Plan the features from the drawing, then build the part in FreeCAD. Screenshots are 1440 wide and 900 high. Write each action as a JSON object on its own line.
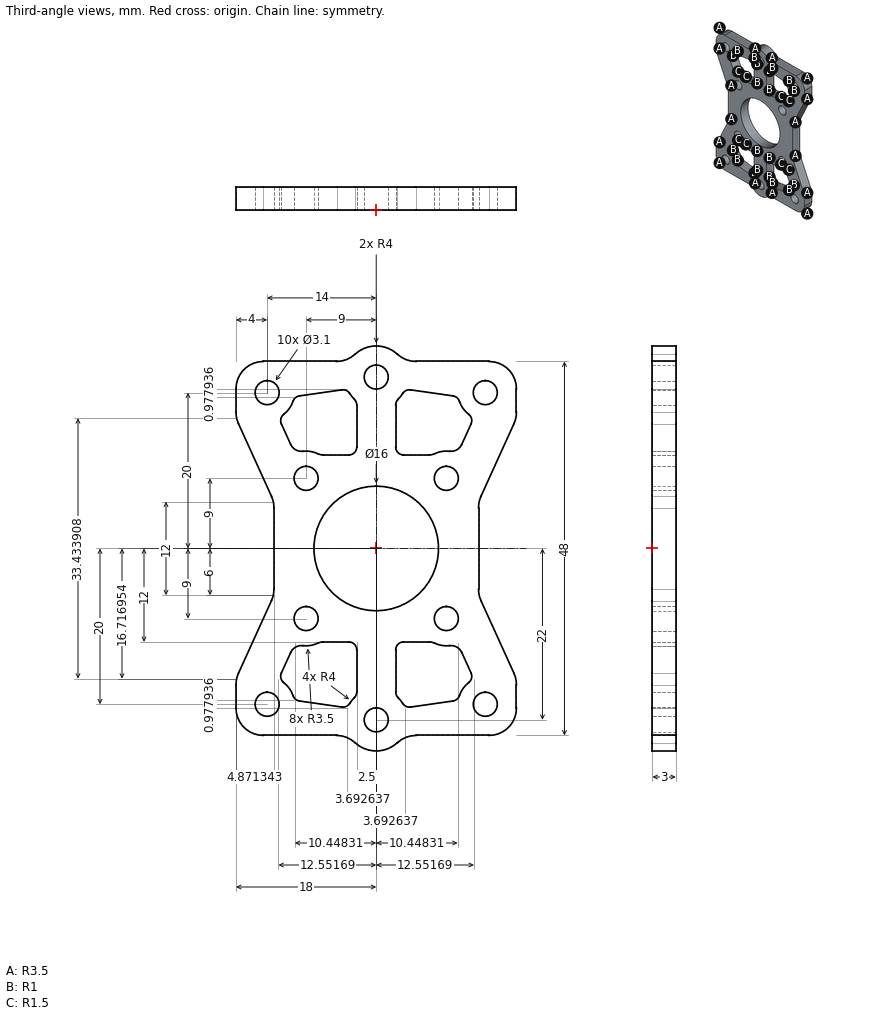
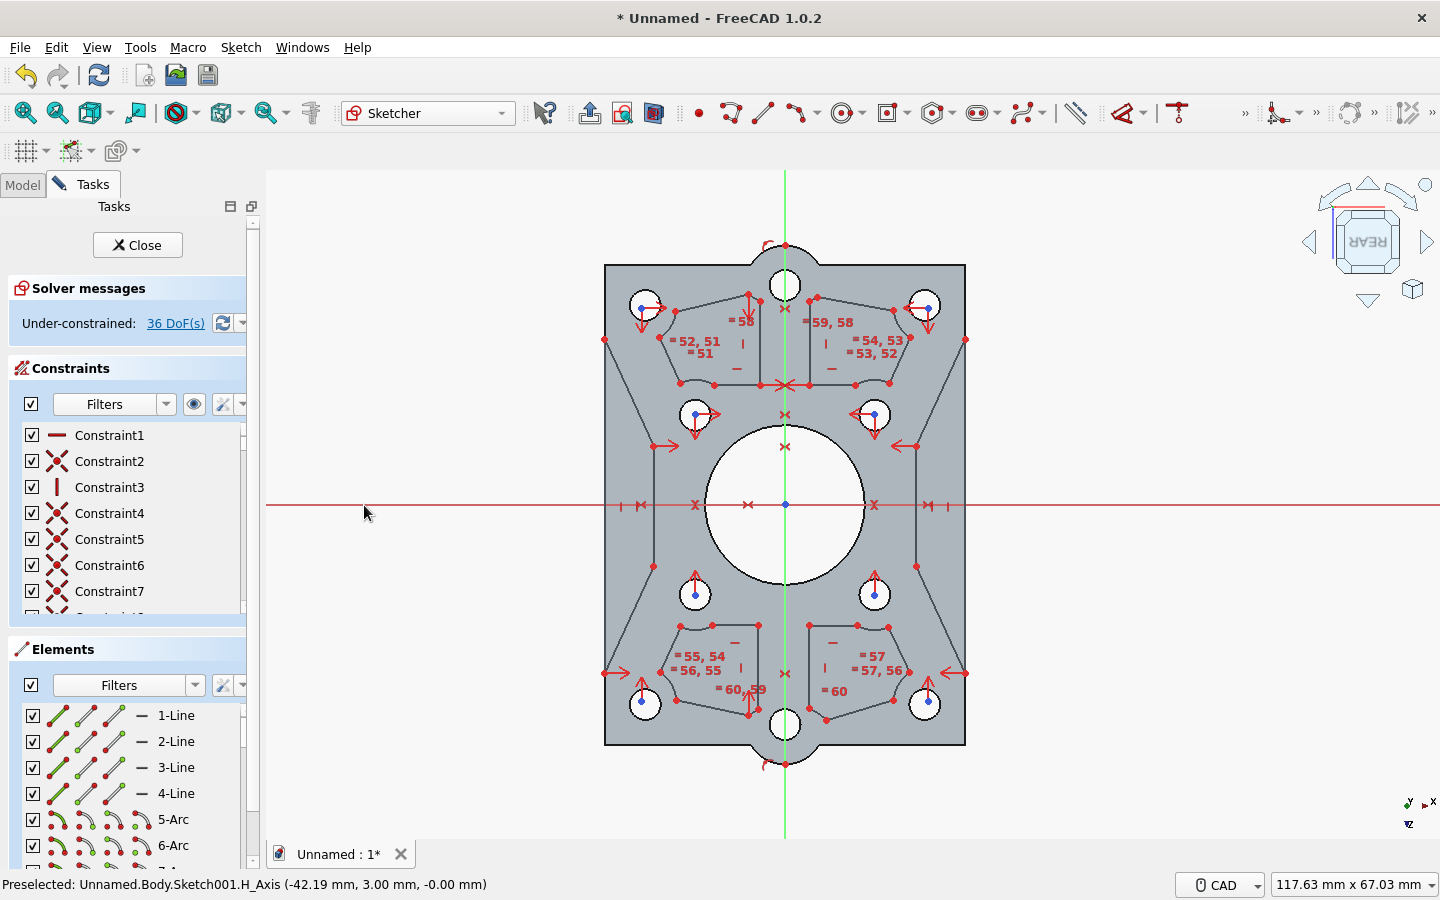
{"action": "left_click", "coordinate": [760, 385]}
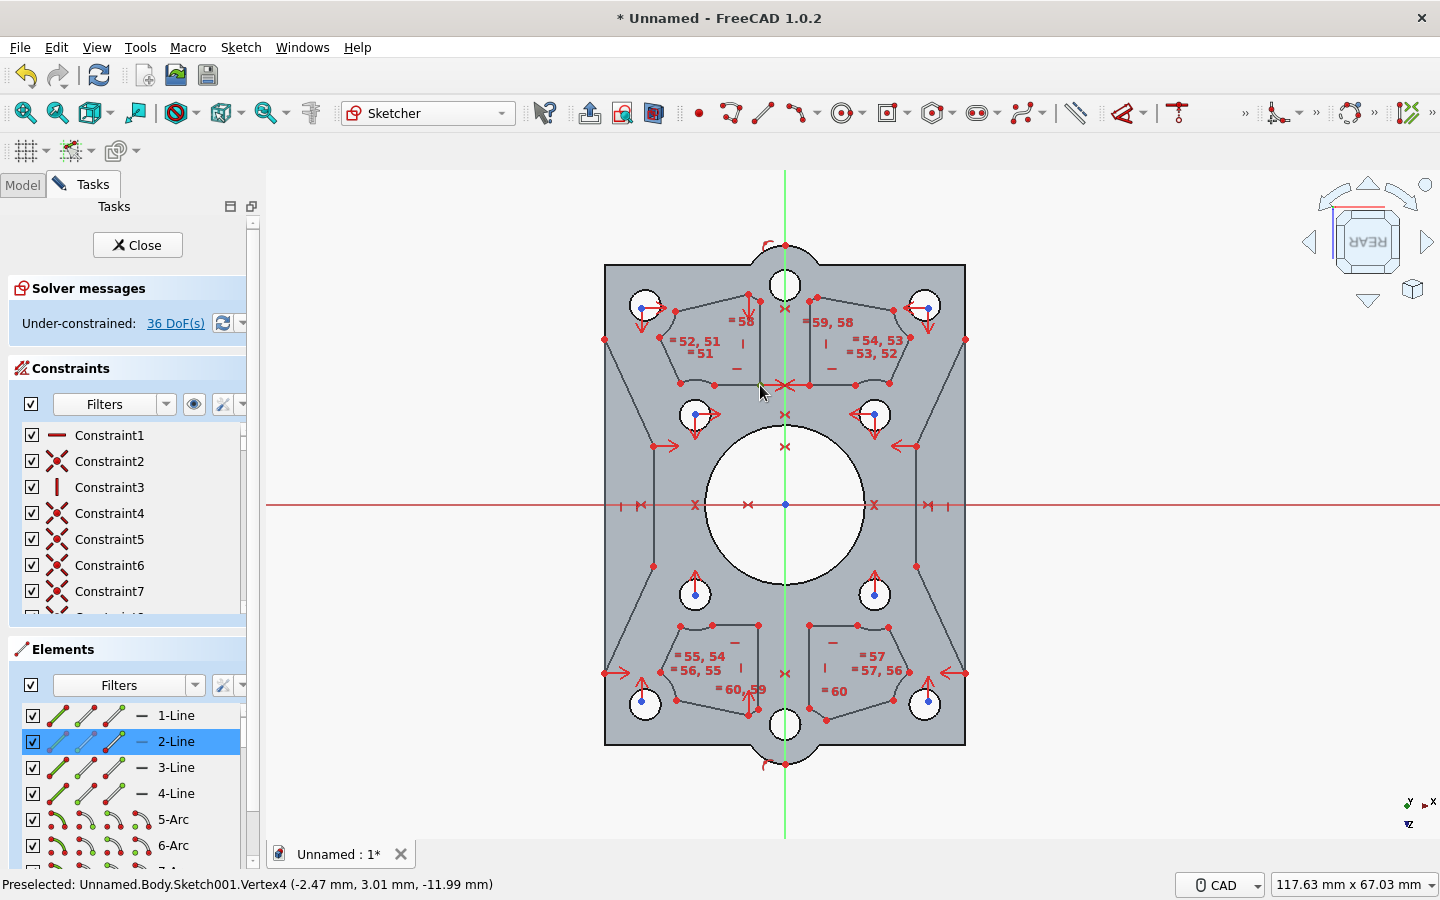
{"action": "left_click", "coordinate": [758, 625]}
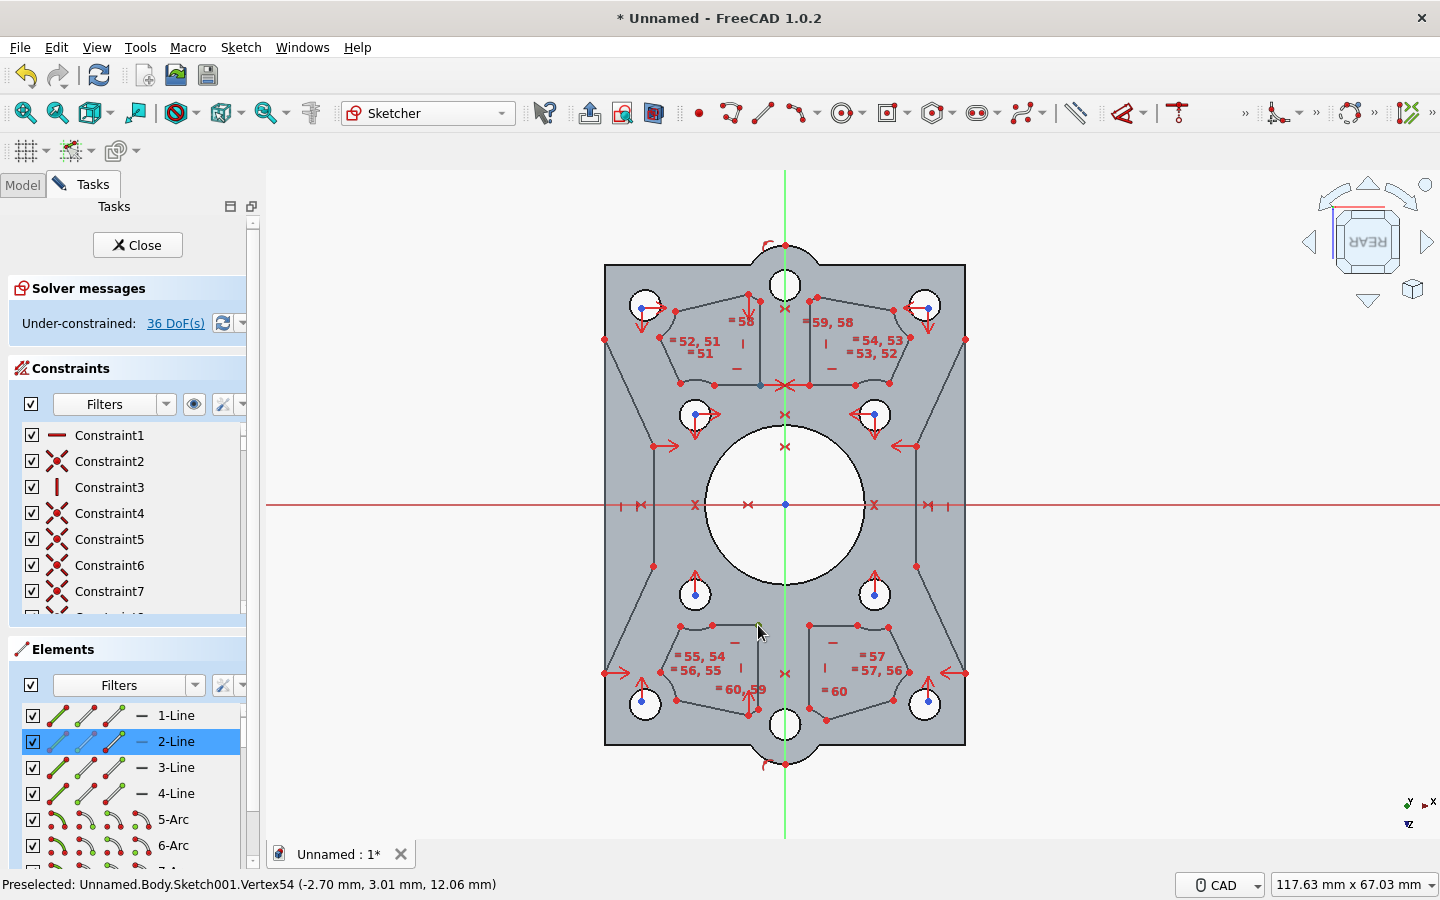
{"action": "left_click", "coordinate": [364, 505]}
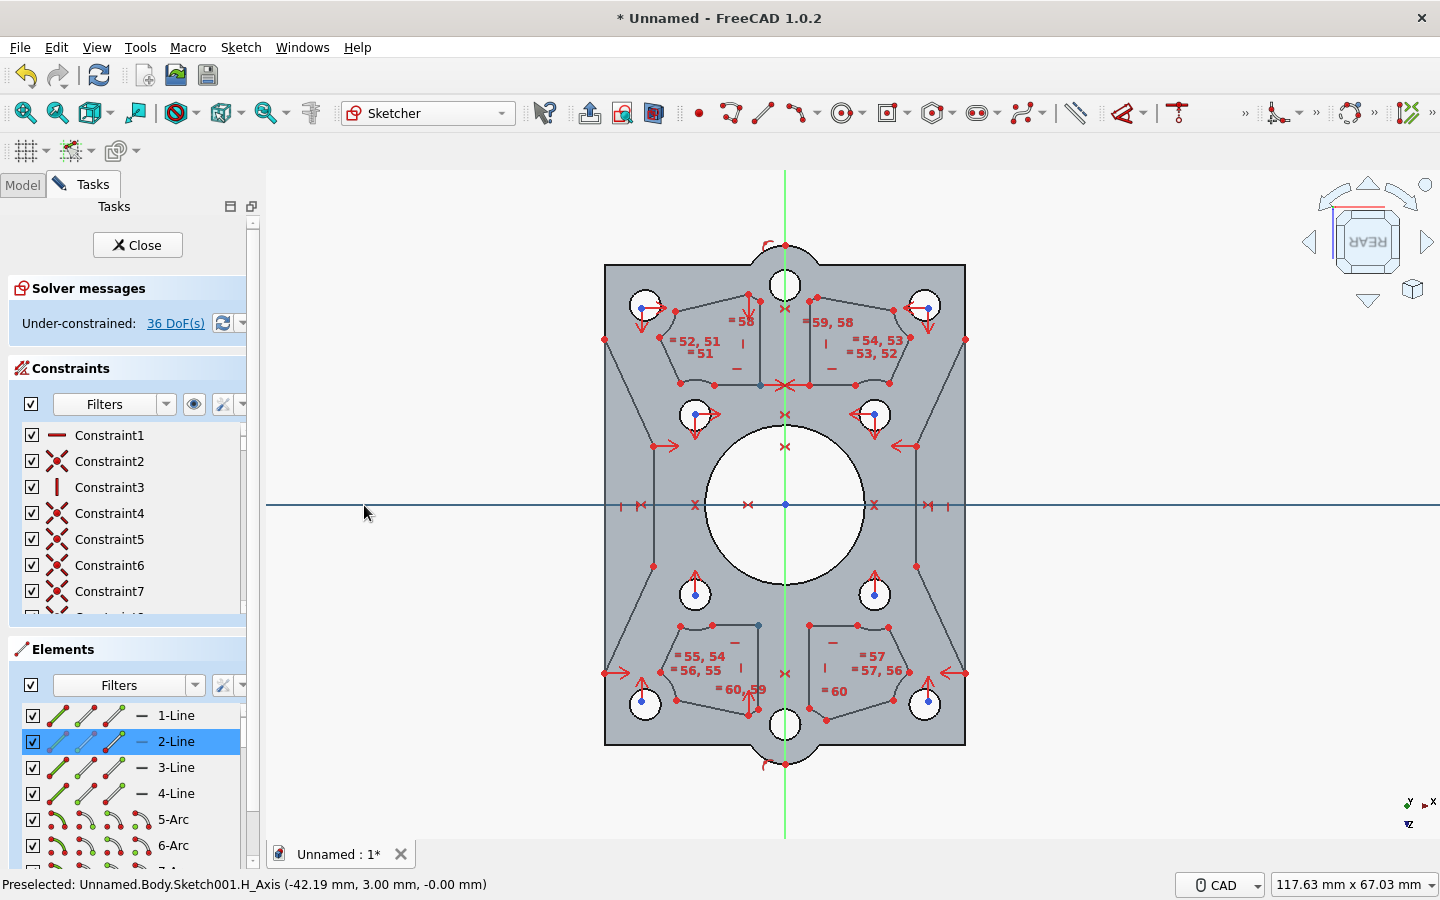
{"action": "key", "text": "s"}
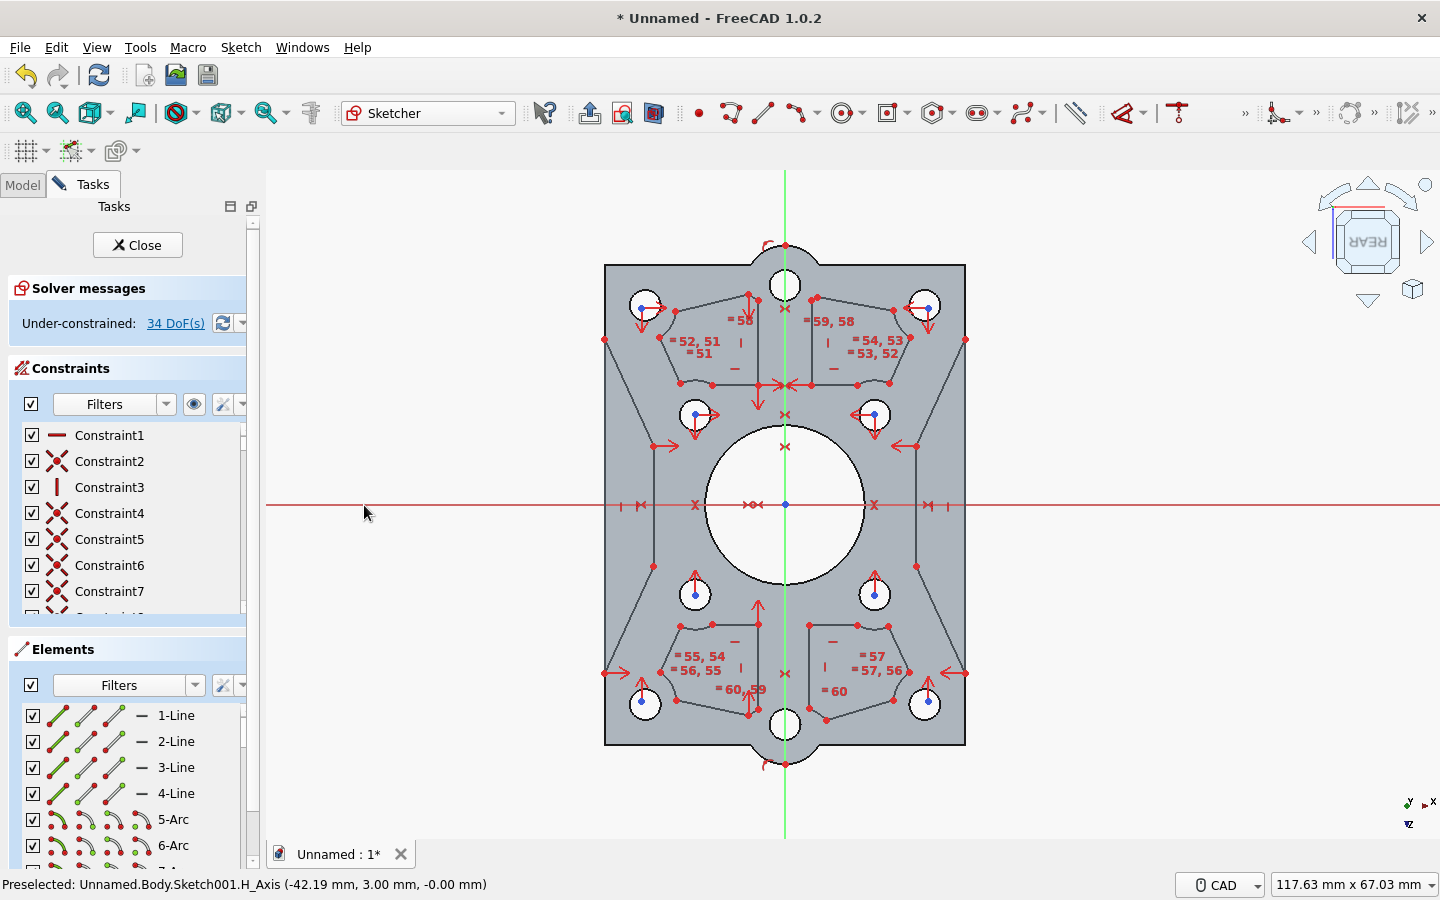
{"action": "left_click", "coordinate": [812, 385]}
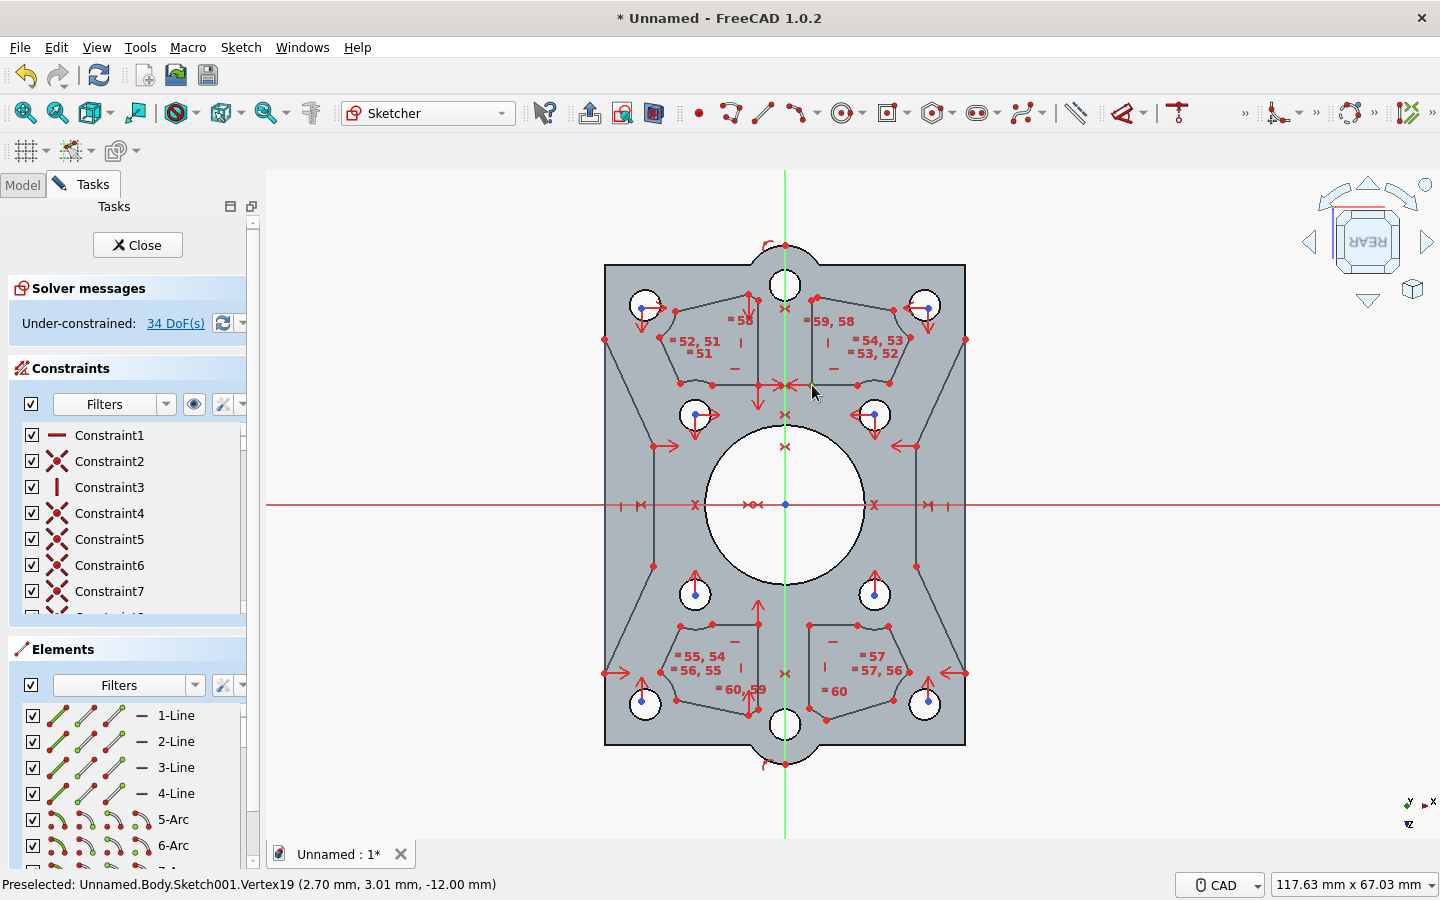
{"action": "left_click", "coordinate": [809, 625]}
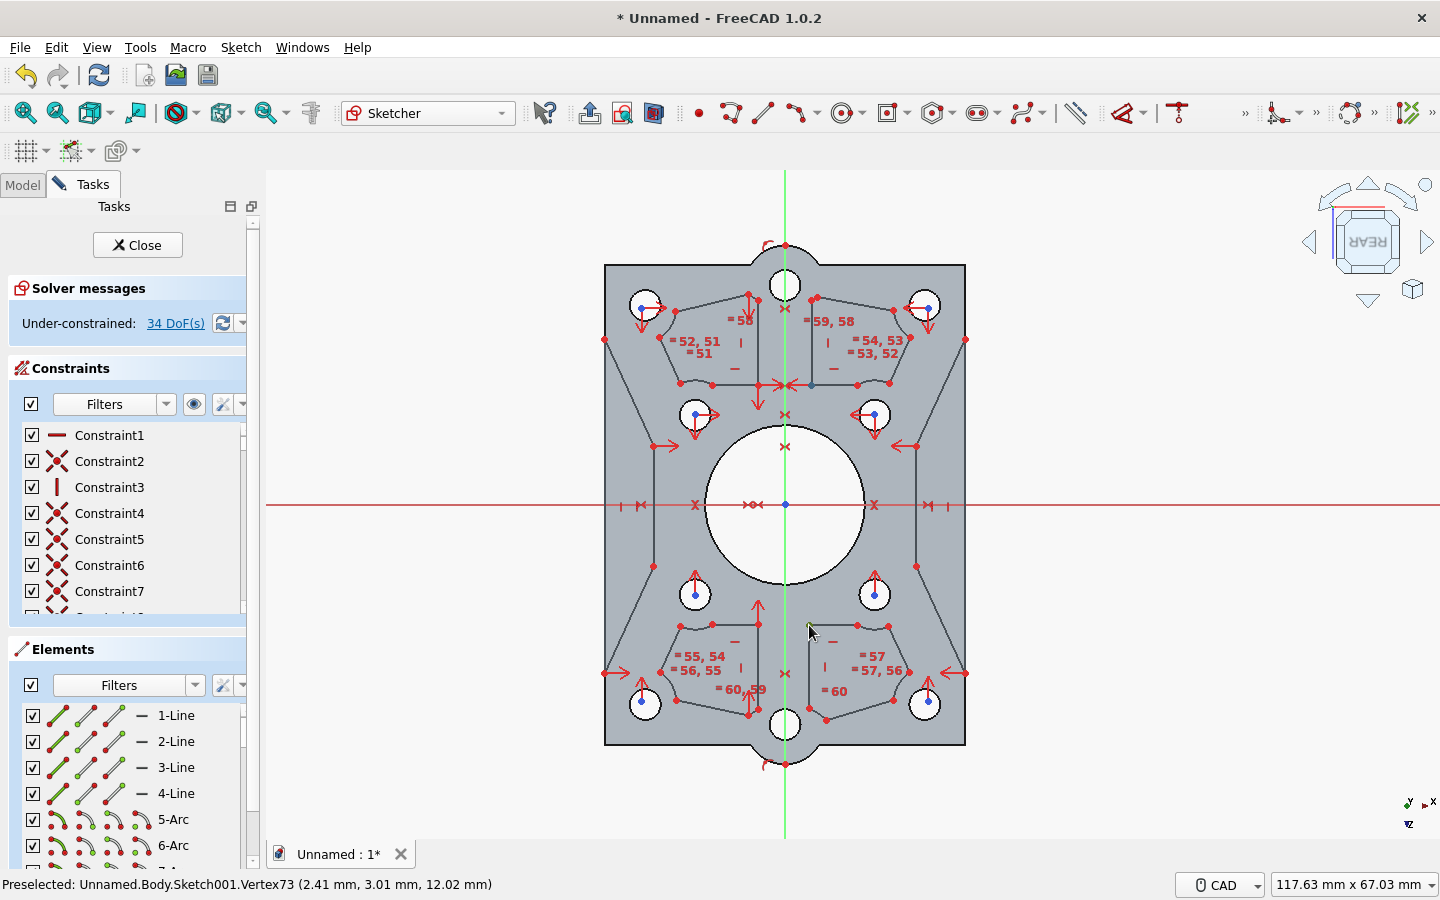
{"action": "left_click", "coordinate": [364, 505]}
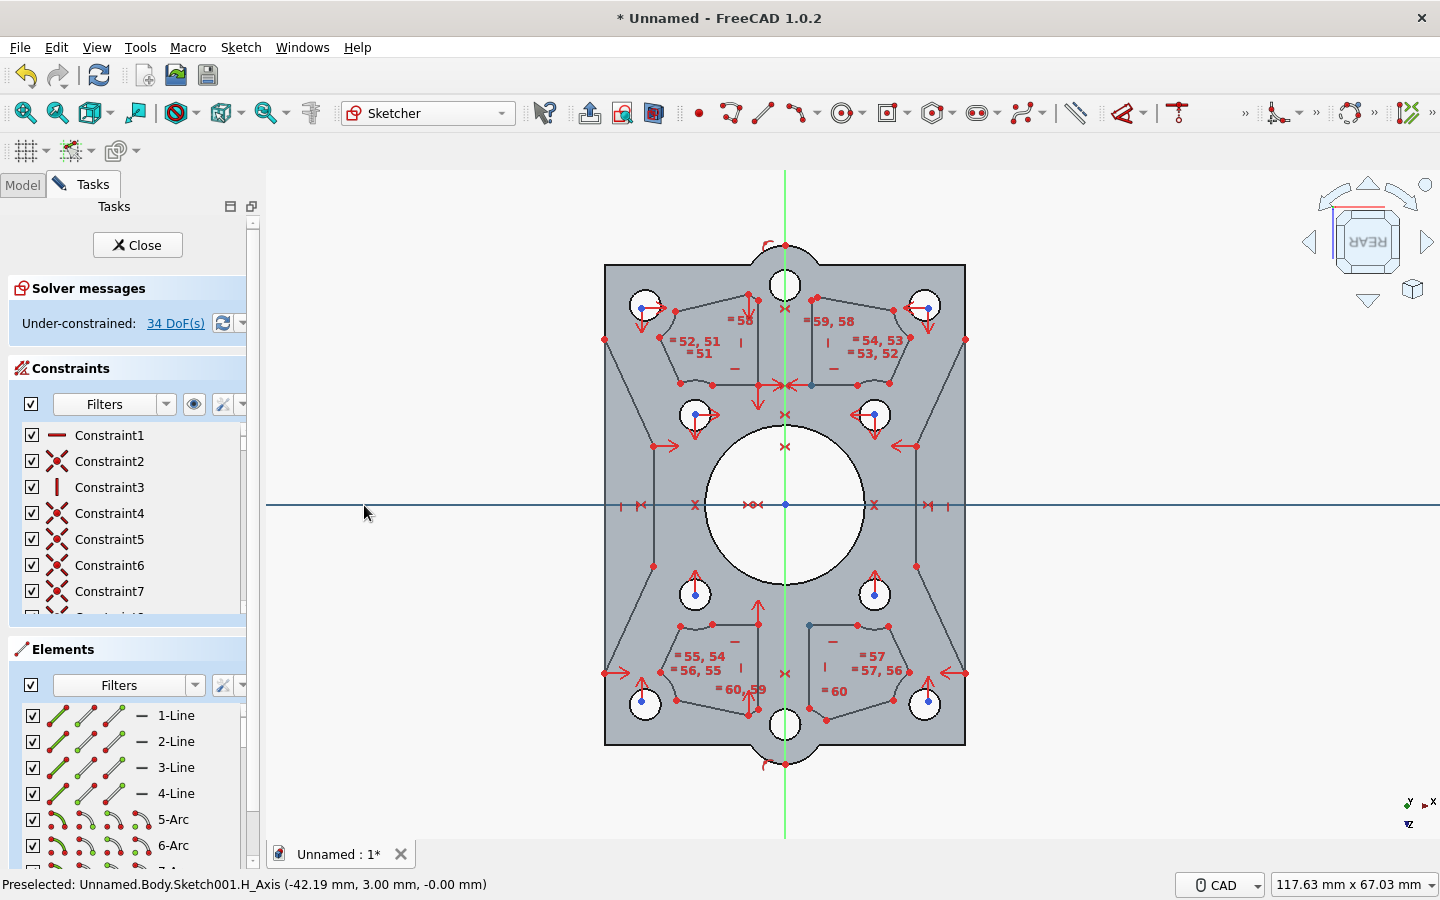
{"action": "key", "text": "s"}